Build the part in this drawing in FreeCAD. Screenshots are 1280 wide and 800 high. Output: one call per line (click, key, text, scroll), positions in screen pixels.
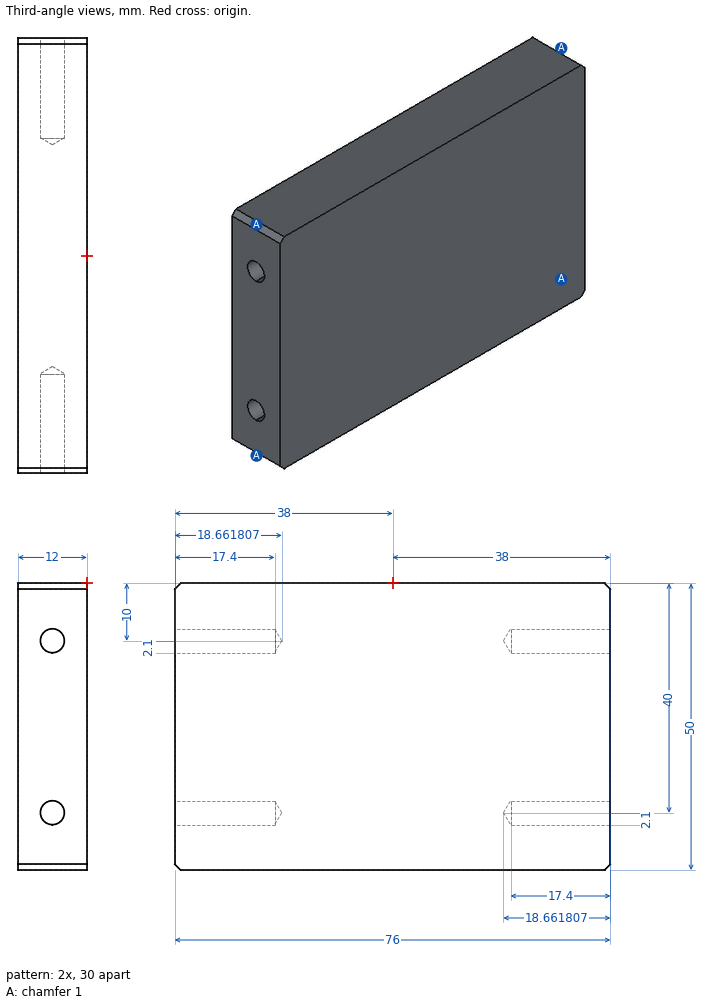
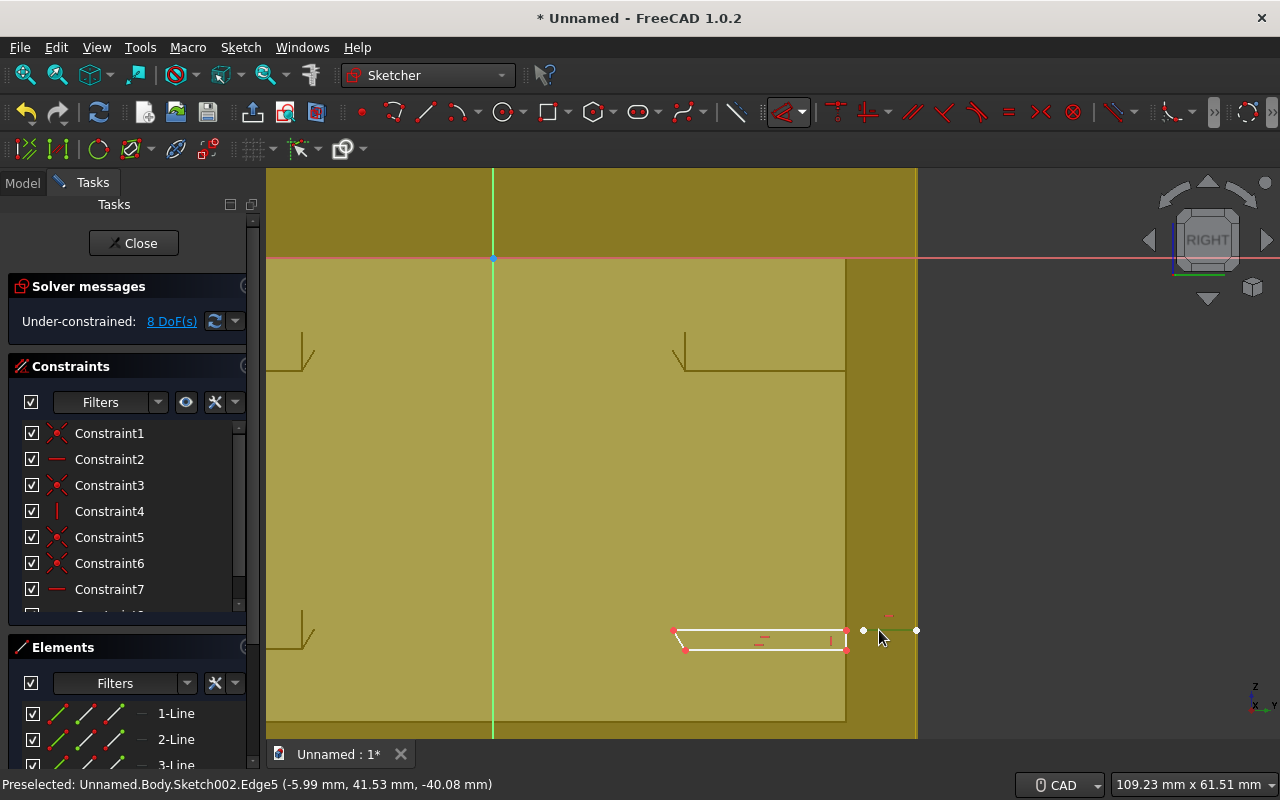
click(738, 112)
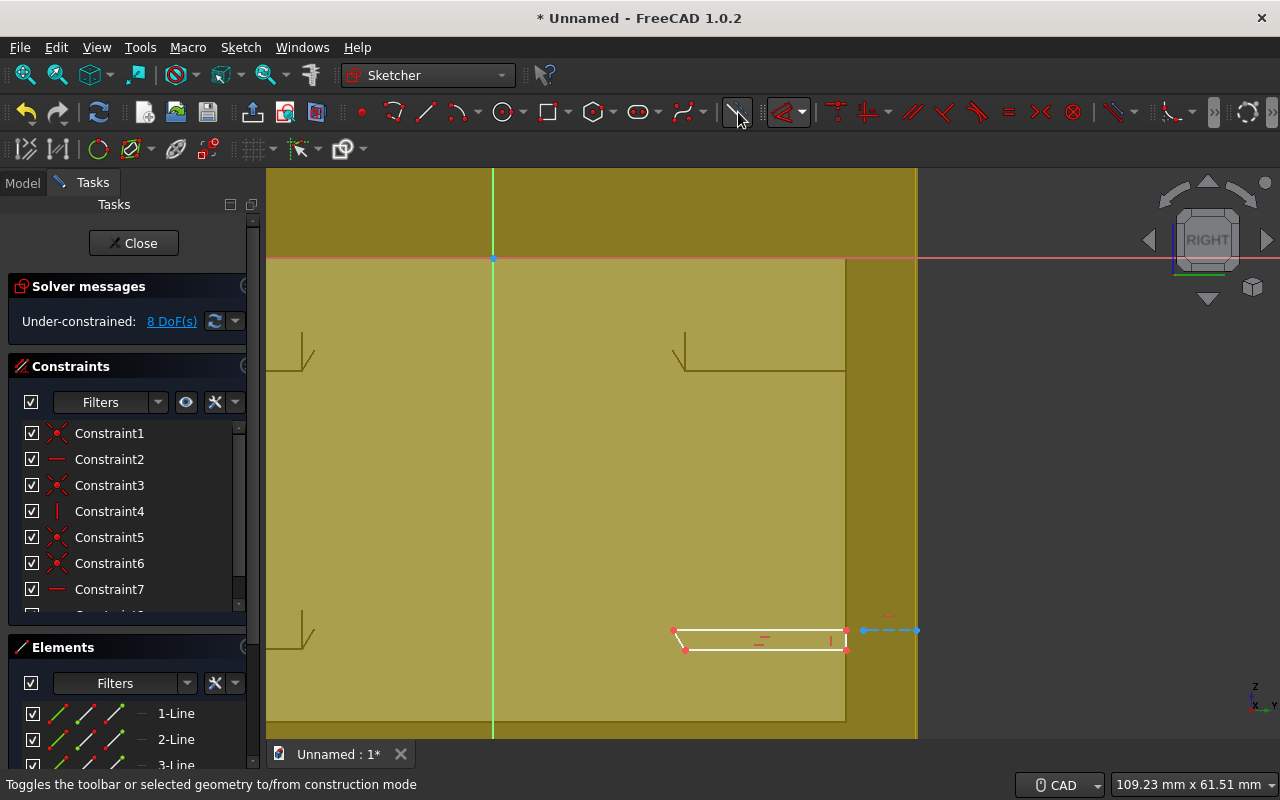
scroll(846, 640, up, 4)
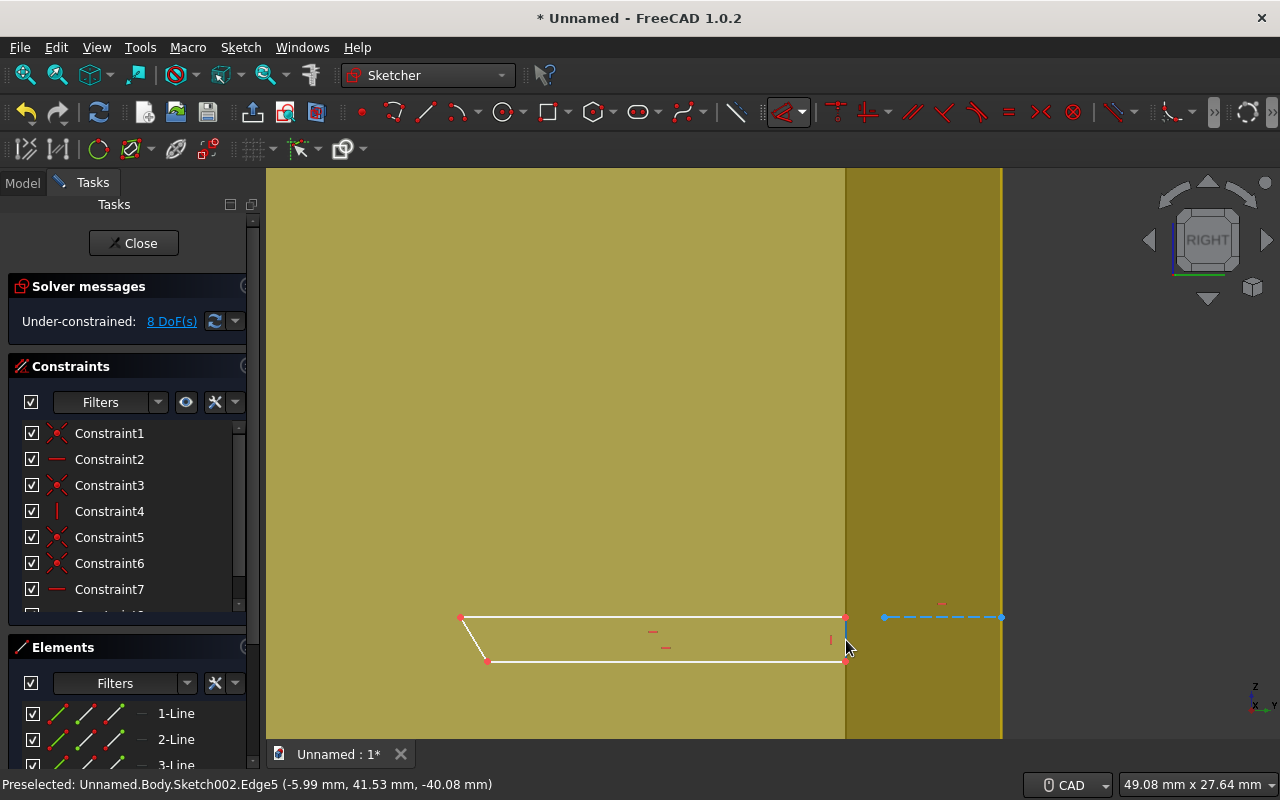
click(846, 640)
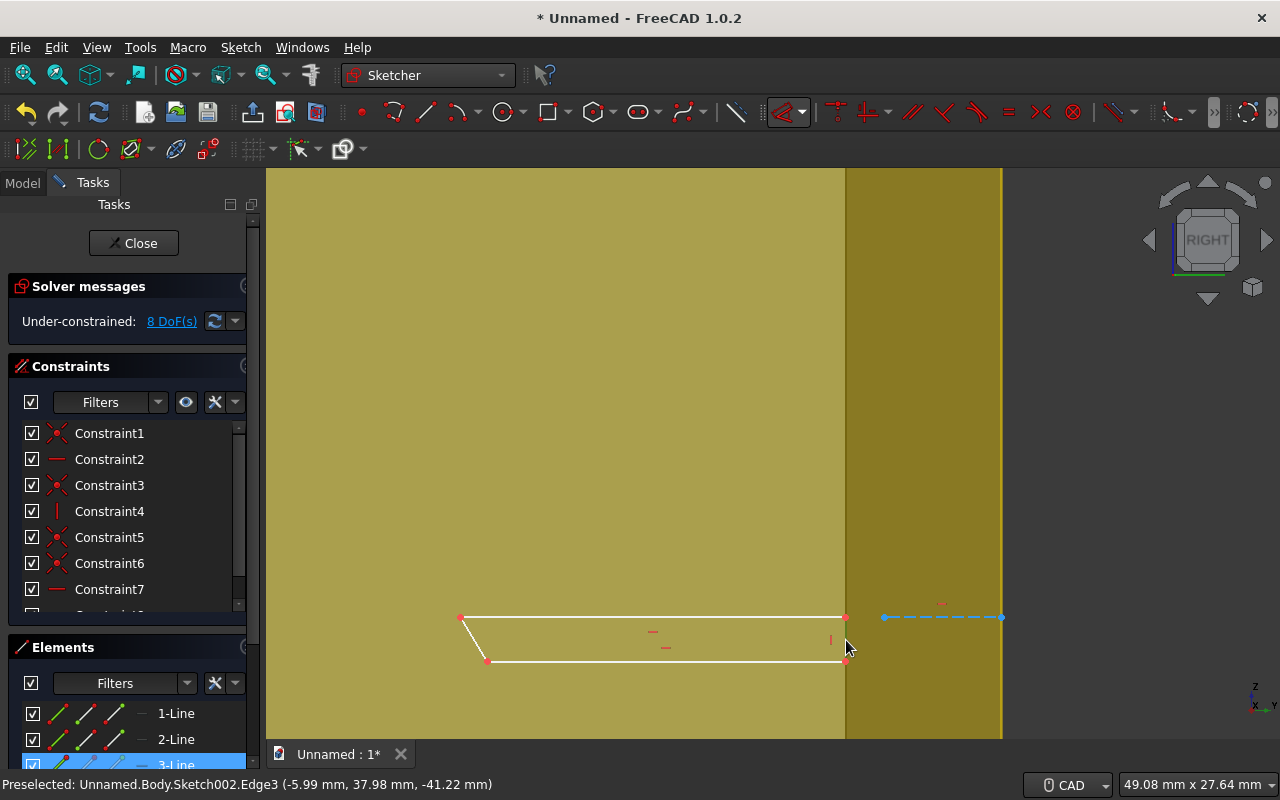
key(i)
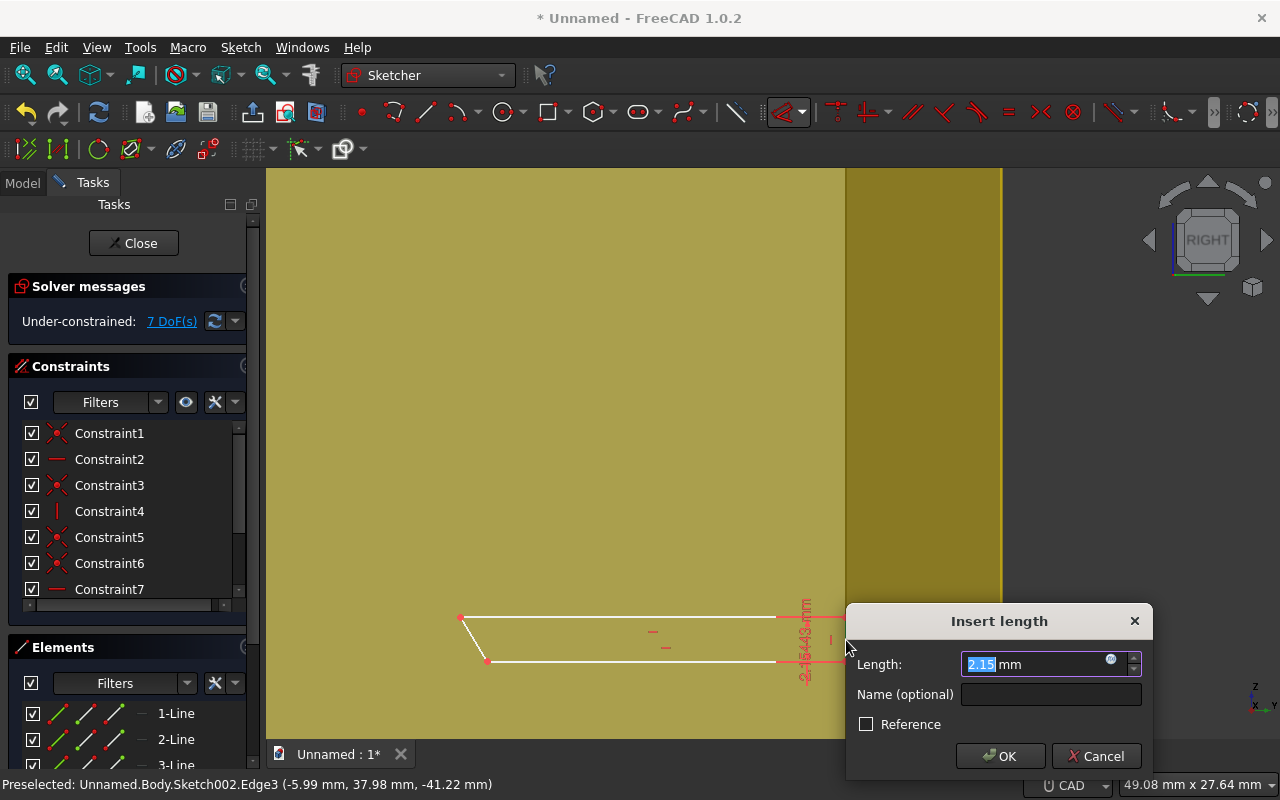
text(2.1)
key(Return)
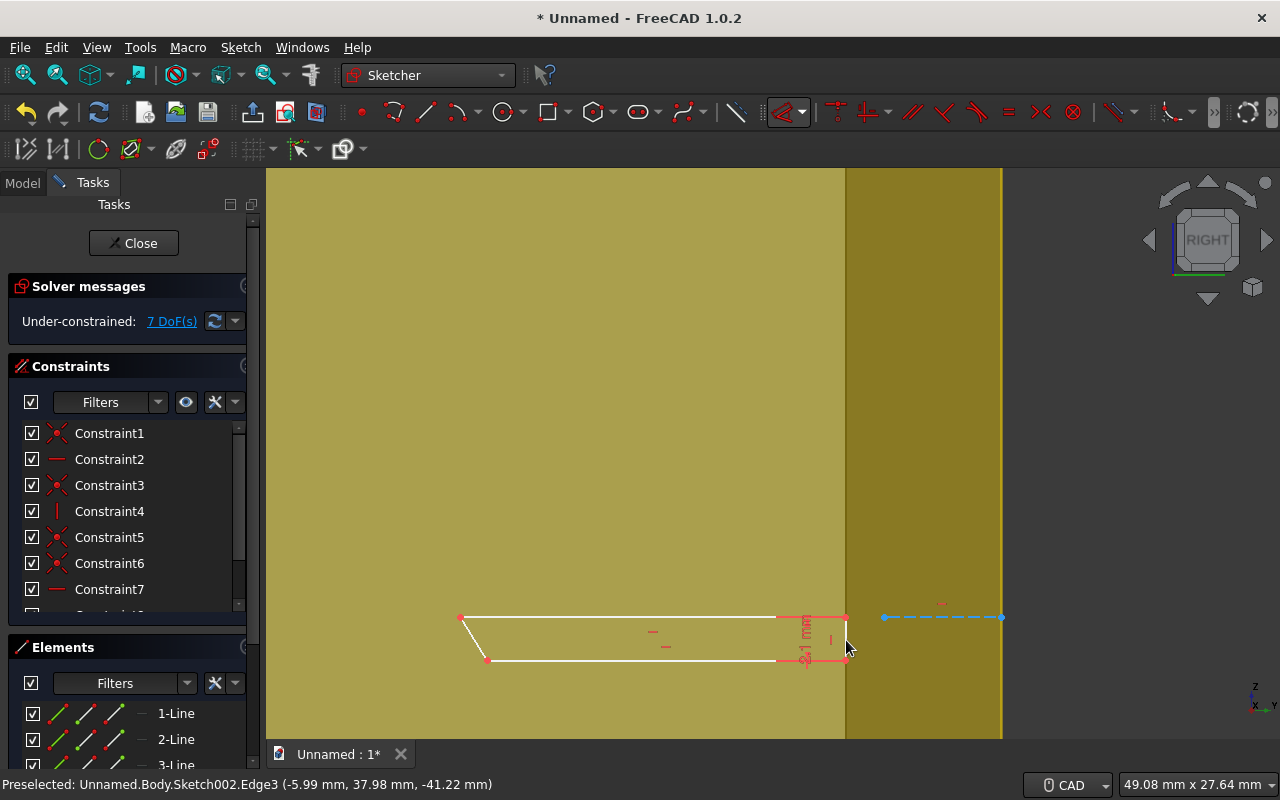
click(461, 617)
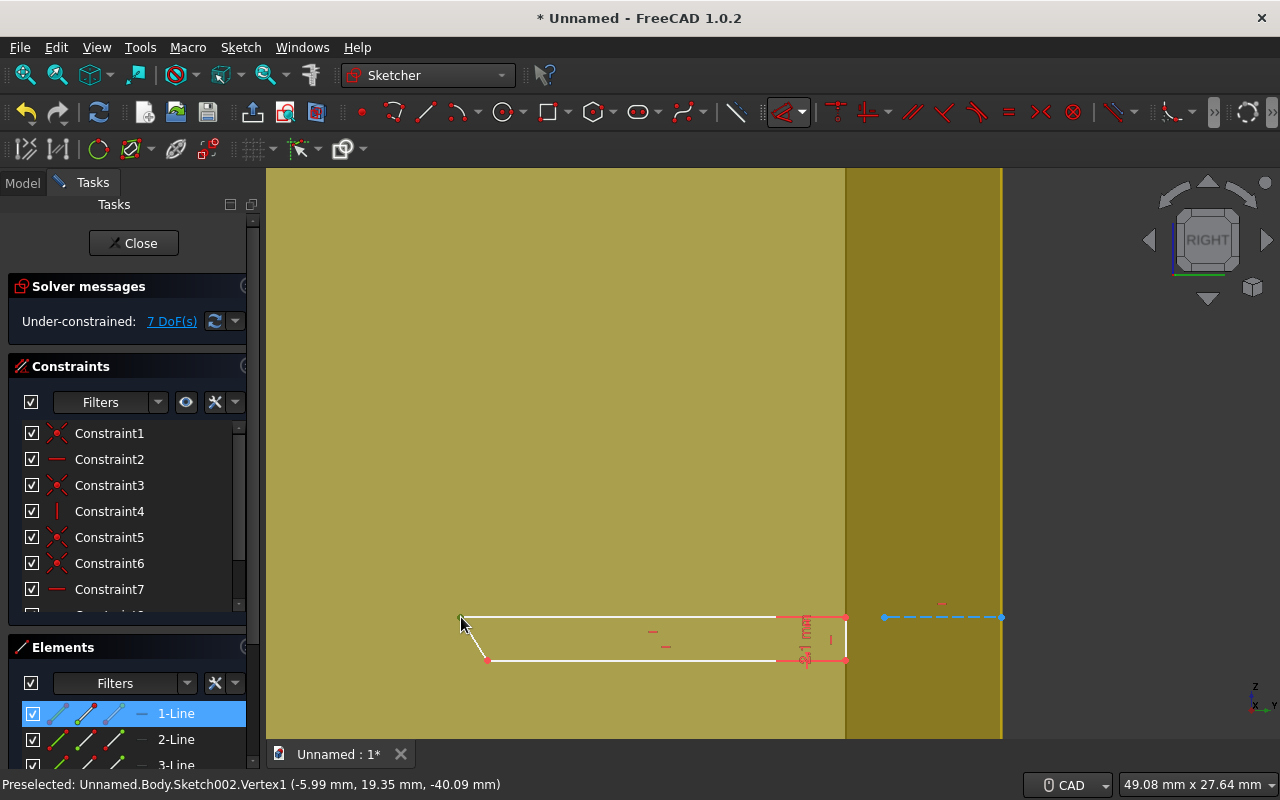
key(i)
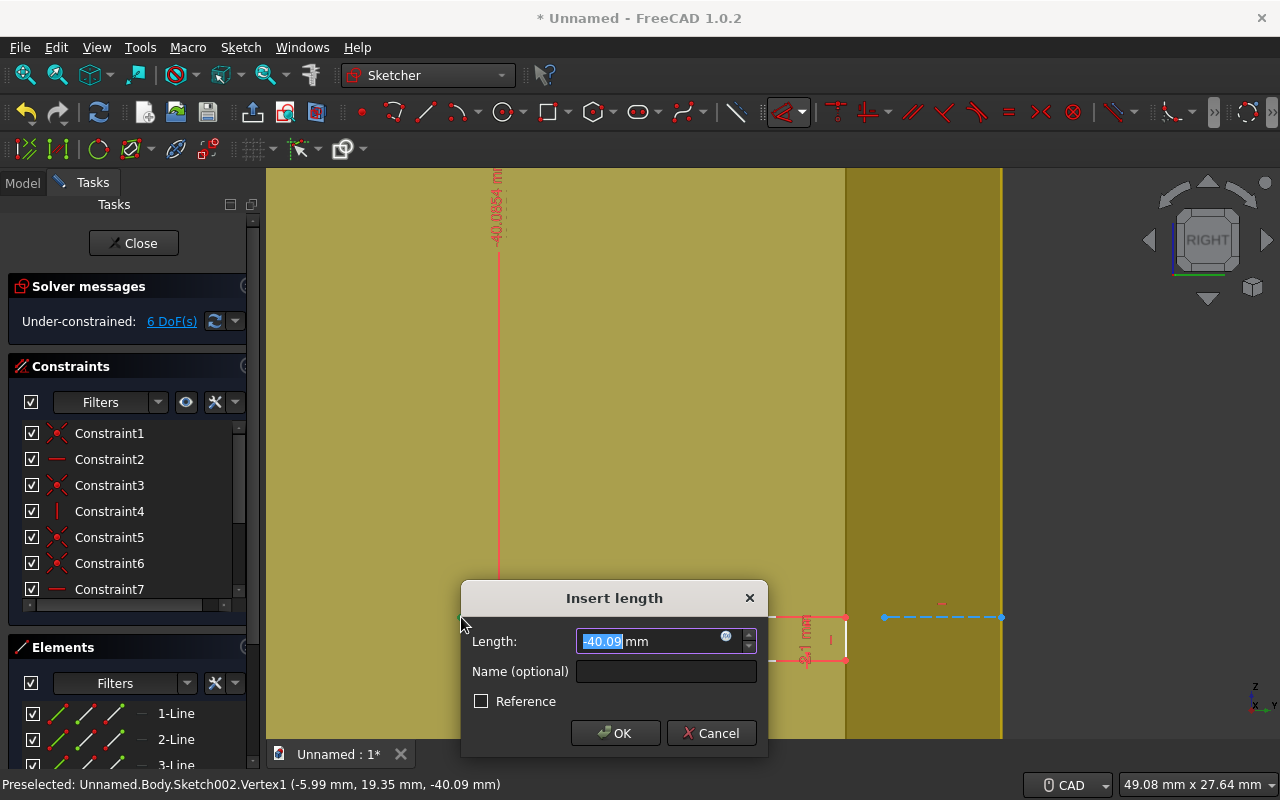
text(-40)
key(Return)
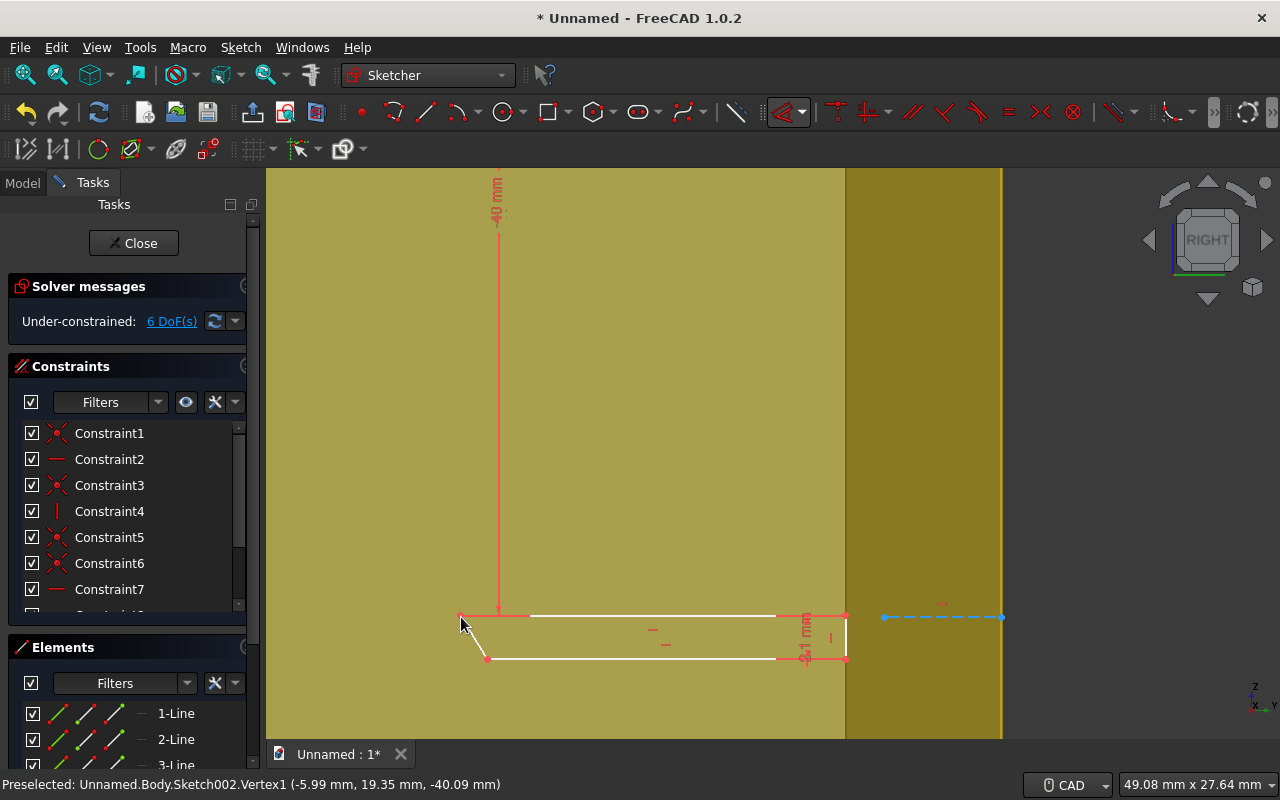
click(846, 659)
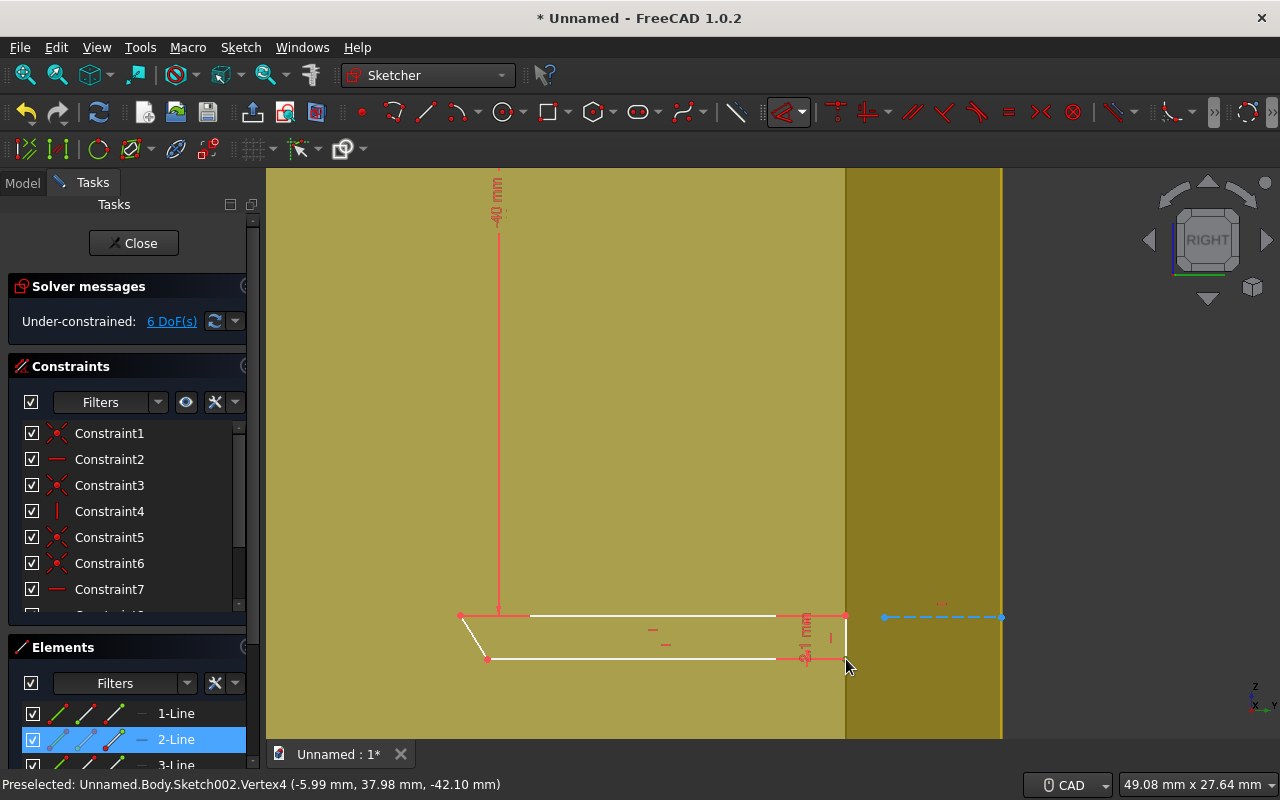
click(804, 112)